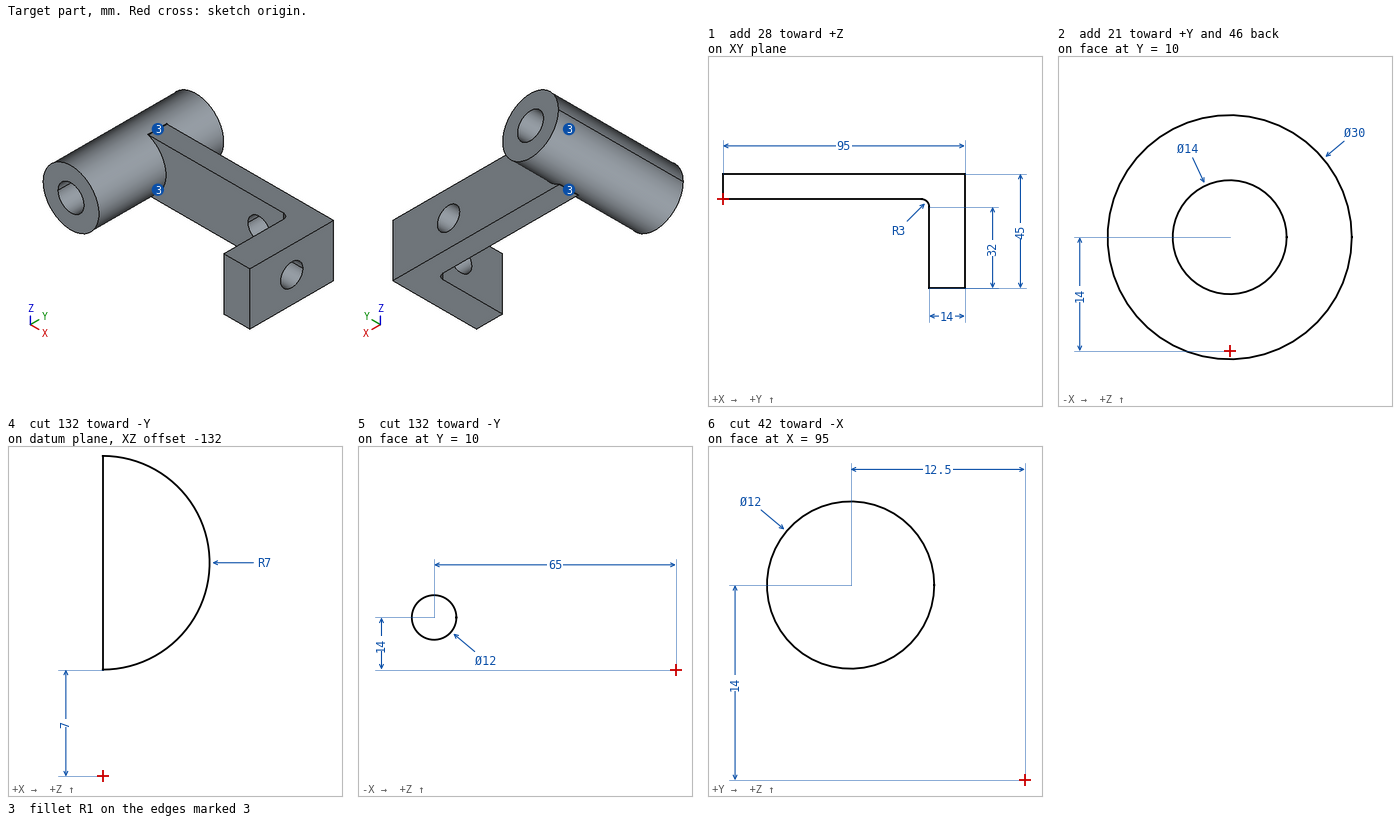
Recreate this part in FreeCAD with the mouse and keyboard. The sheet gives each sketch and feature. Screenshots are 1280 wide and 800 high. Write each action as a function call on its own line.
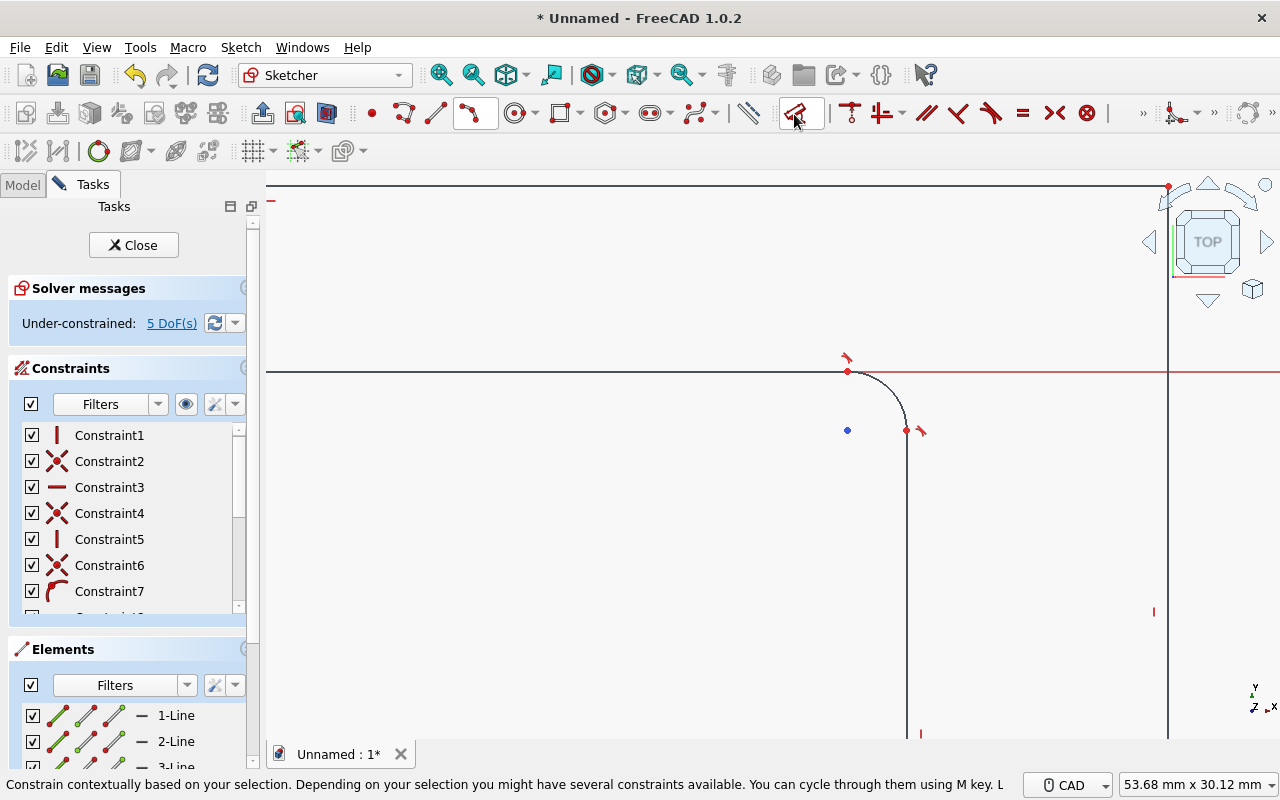
click(900, 404)
click(928, 389)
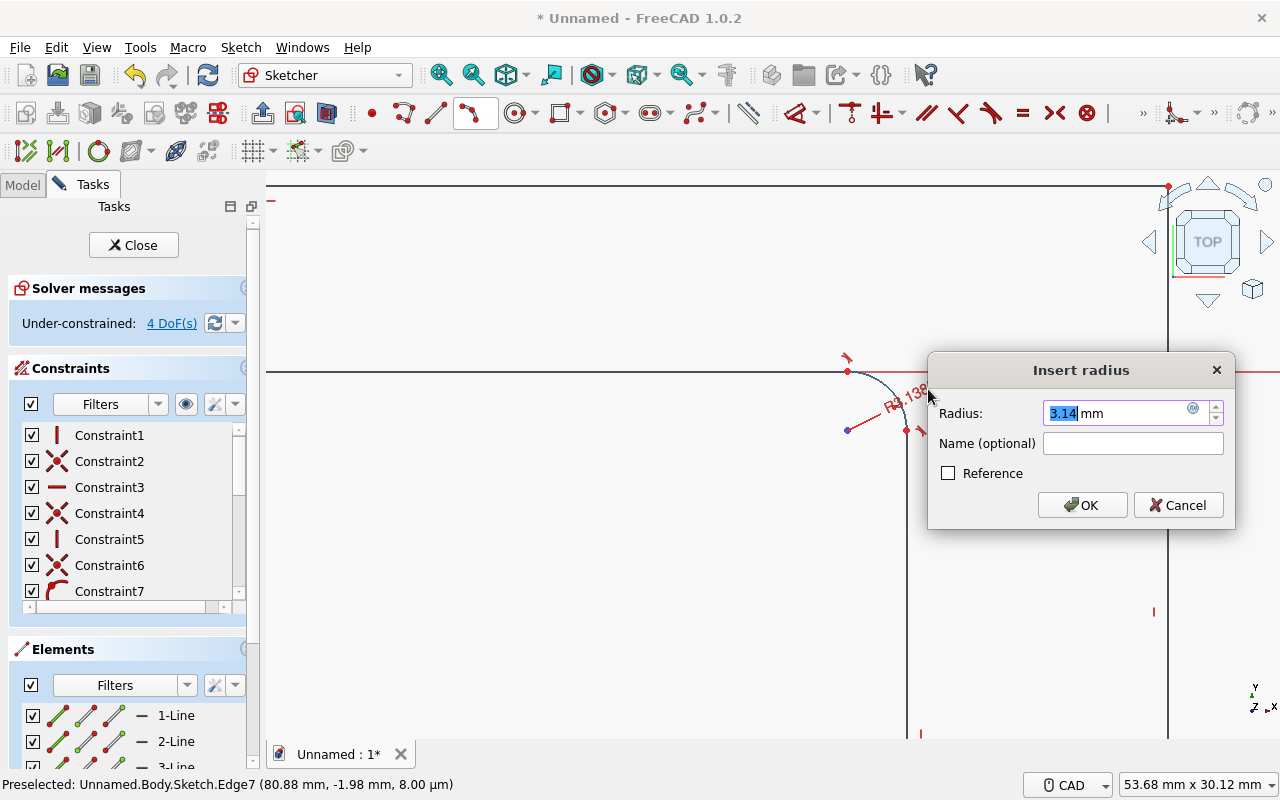
text(3)
key(Return)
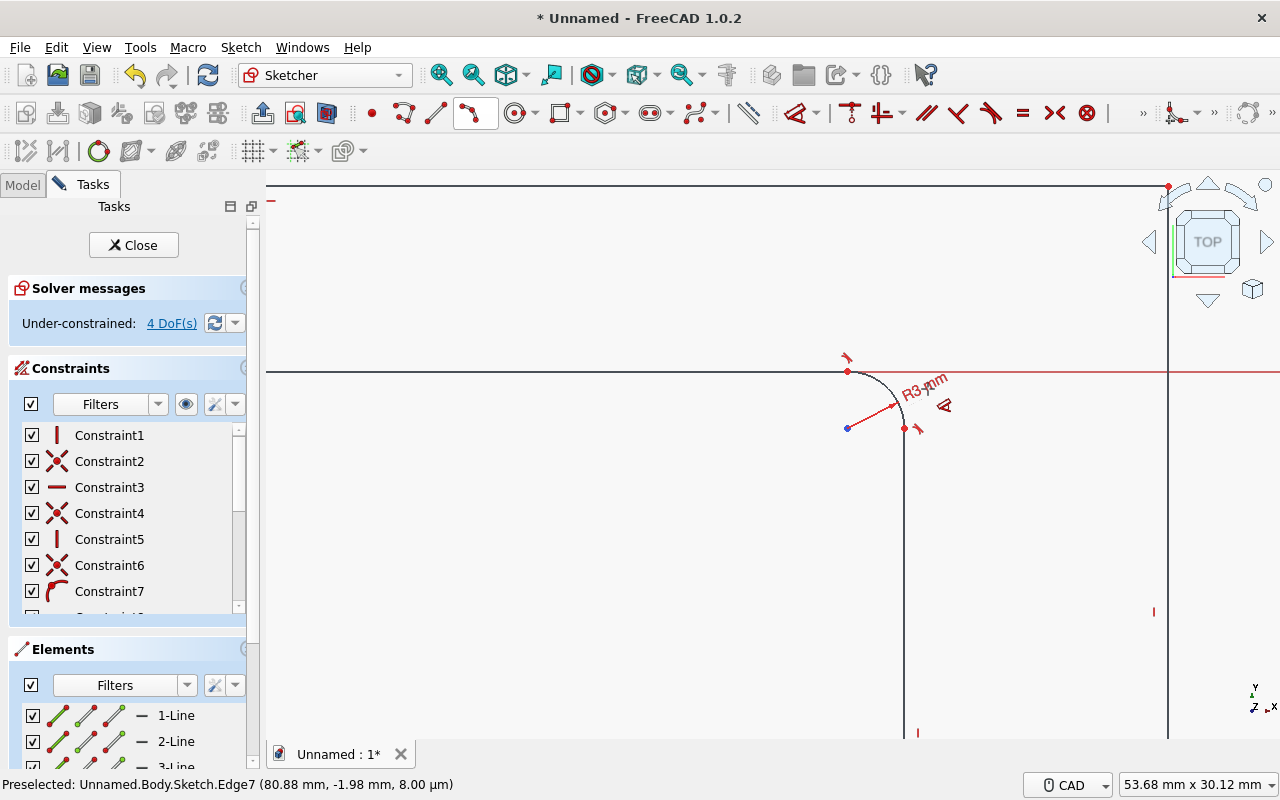
click(904, 611)
click(938, 570)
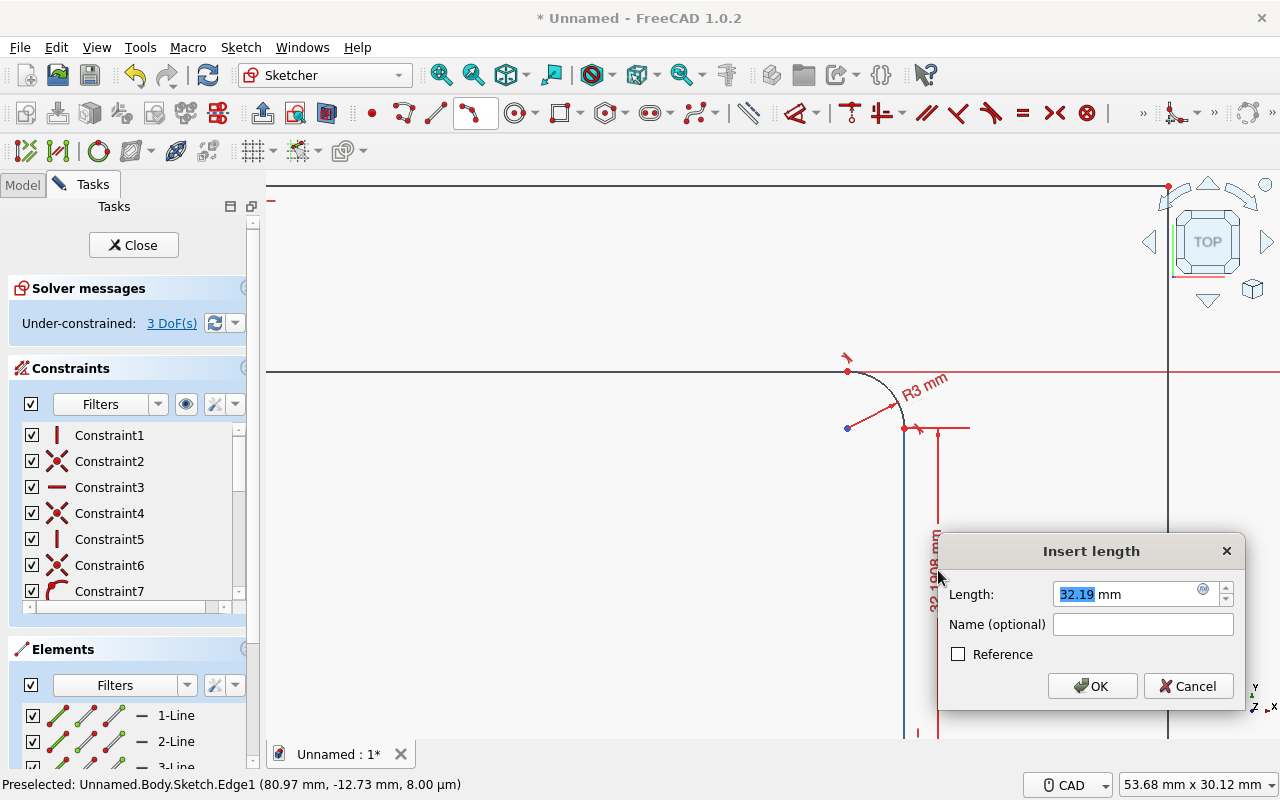
text(32)
key(Return)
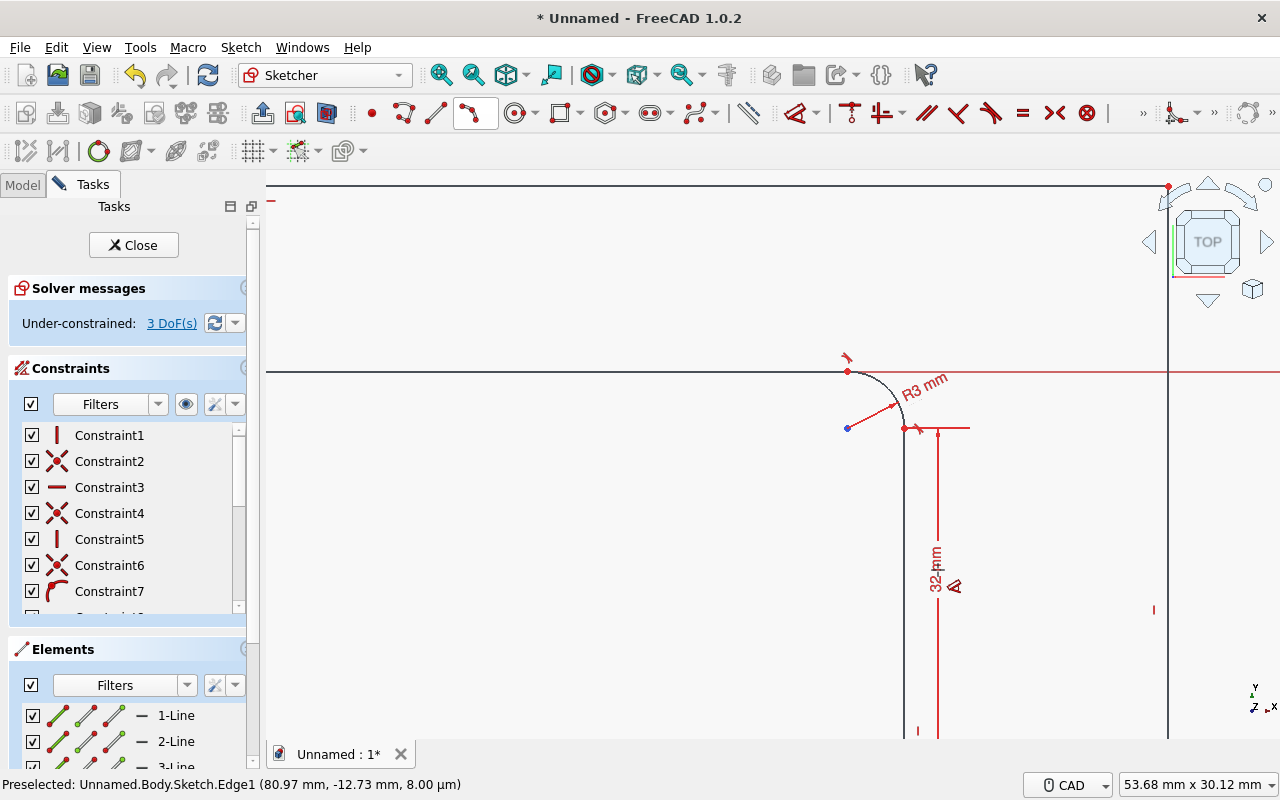
scroll(891, 388, down, 6)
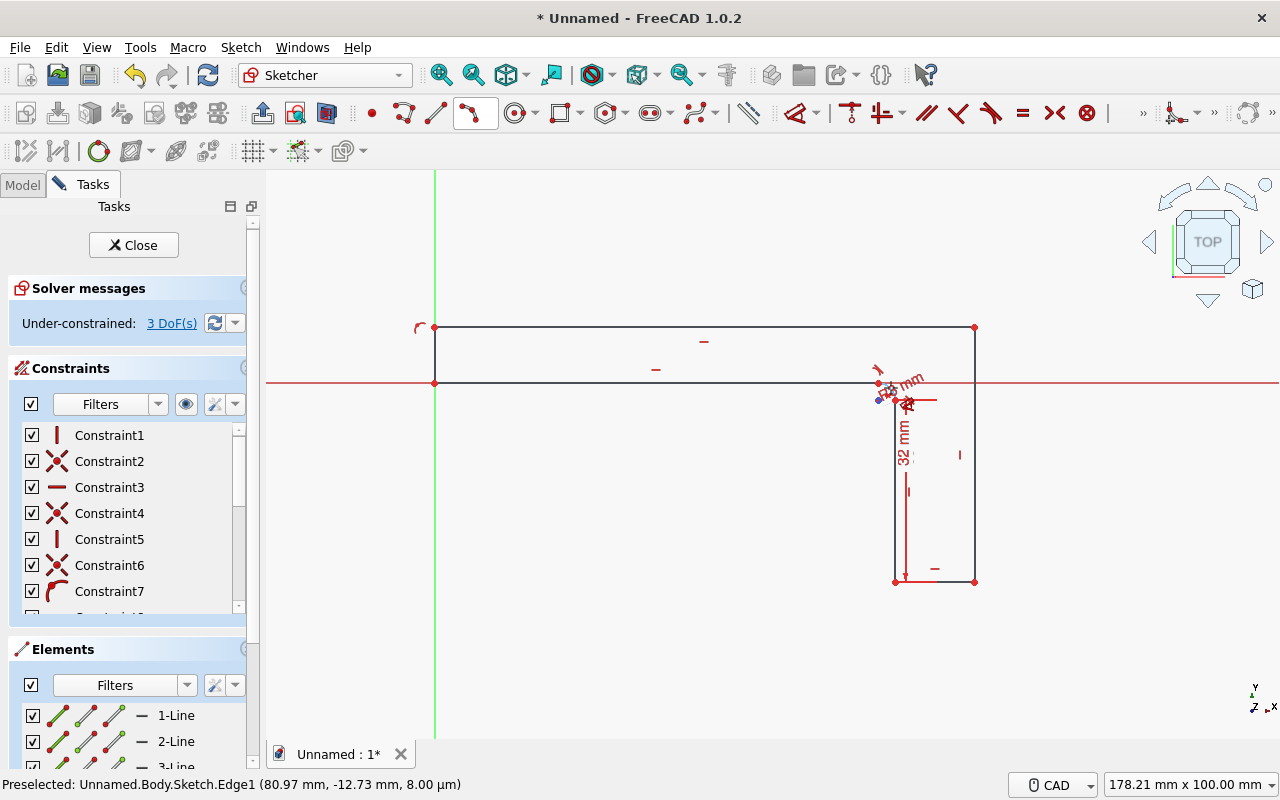
click(919, 582)
click(935, 616)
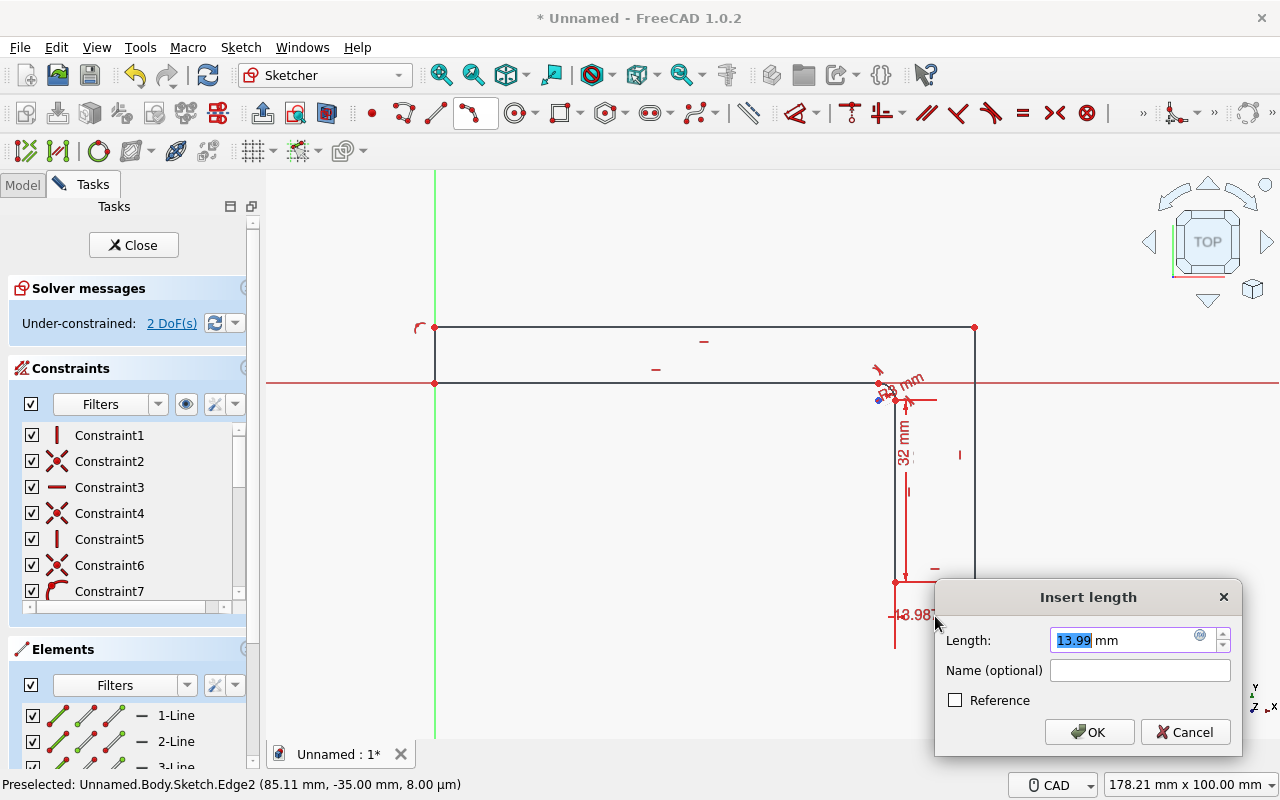
text(14)
key(Return)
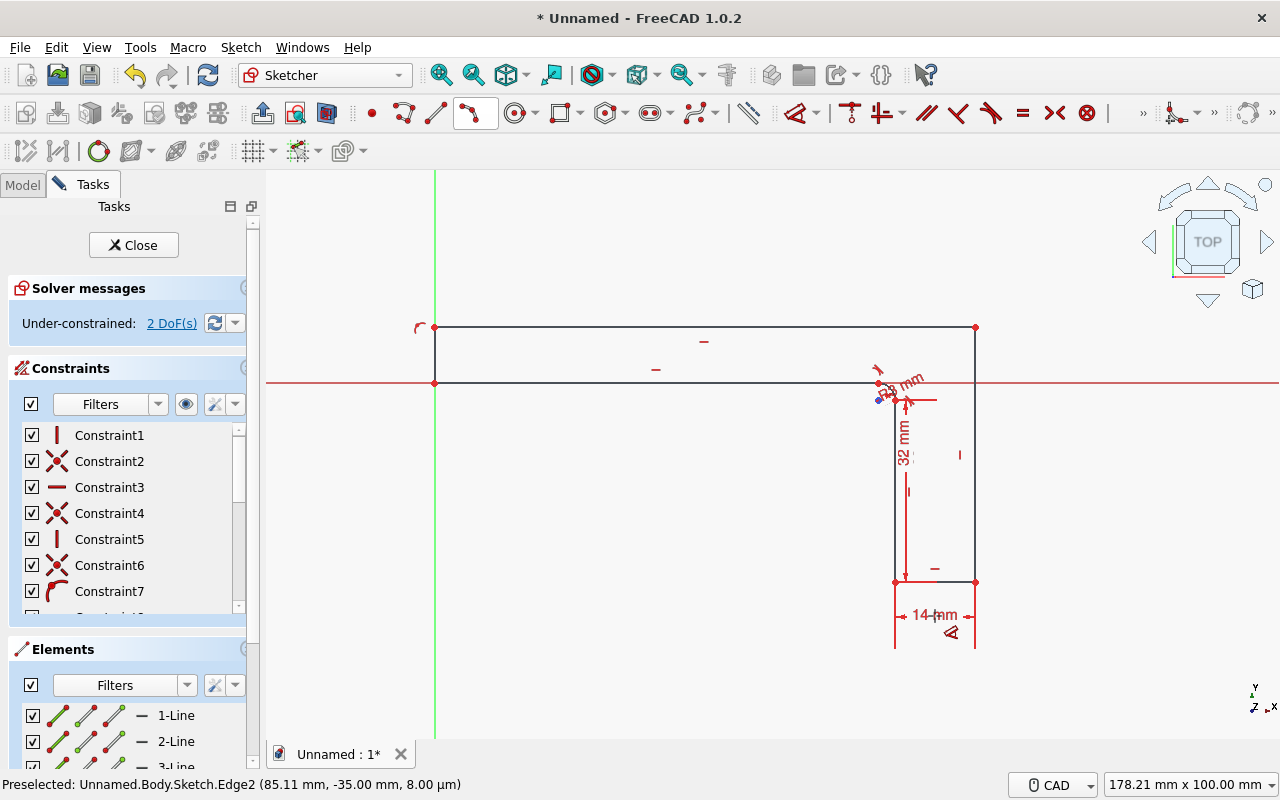
click(975, 506)
click(1009, 455)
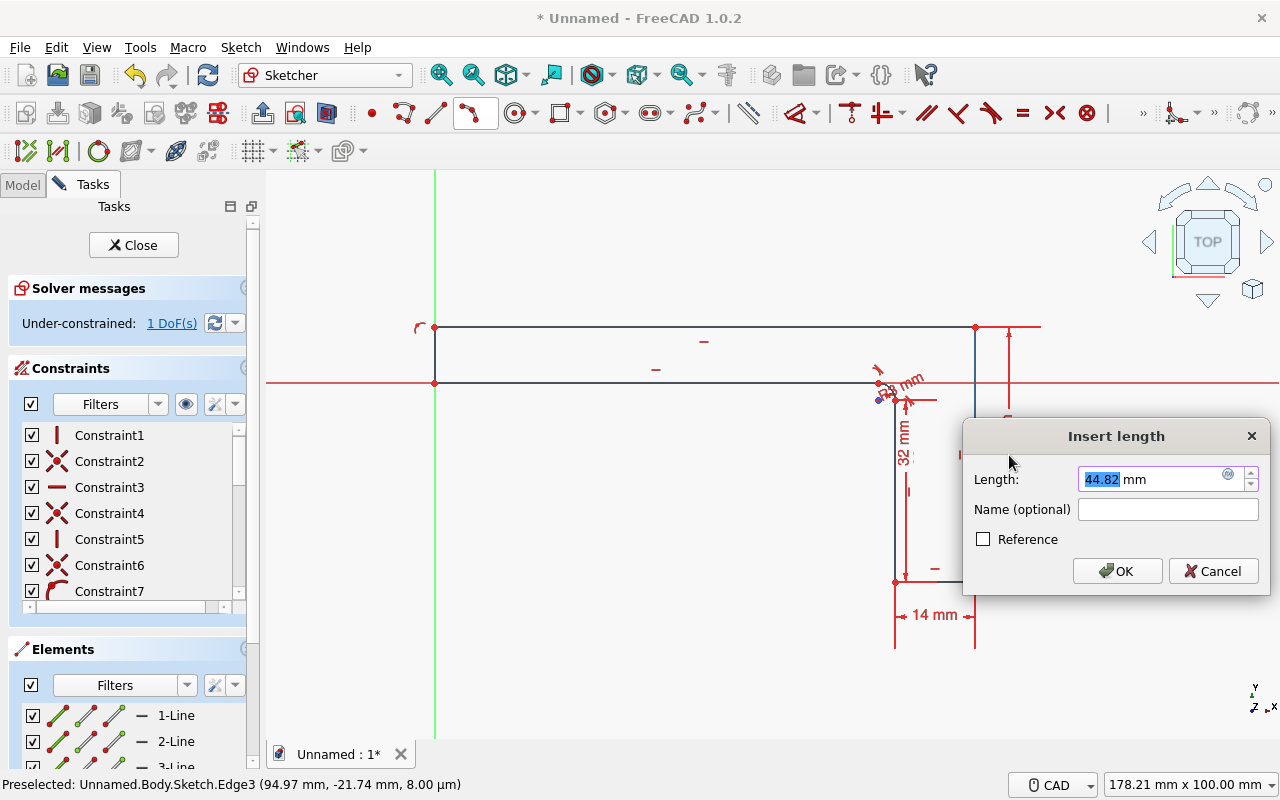
text(45)
key(Return)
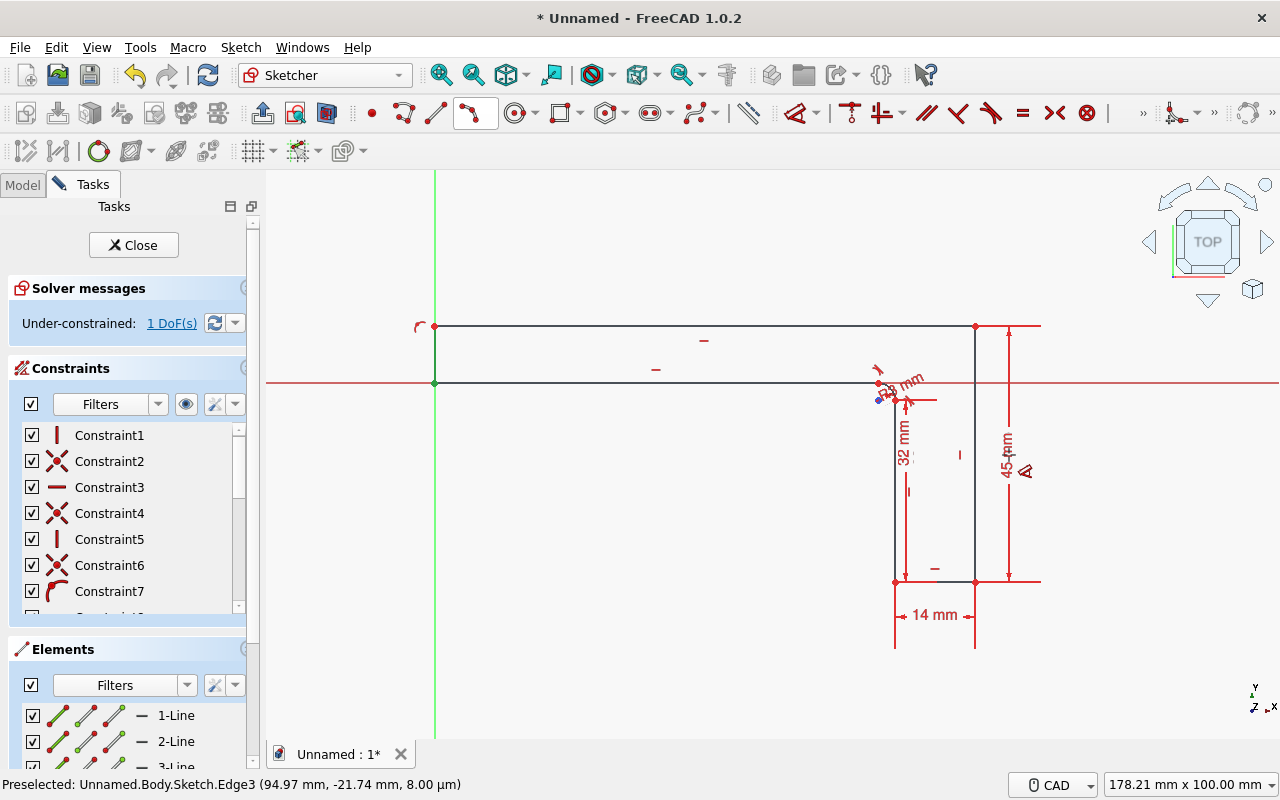
click(813, 326)
click(705, 292)